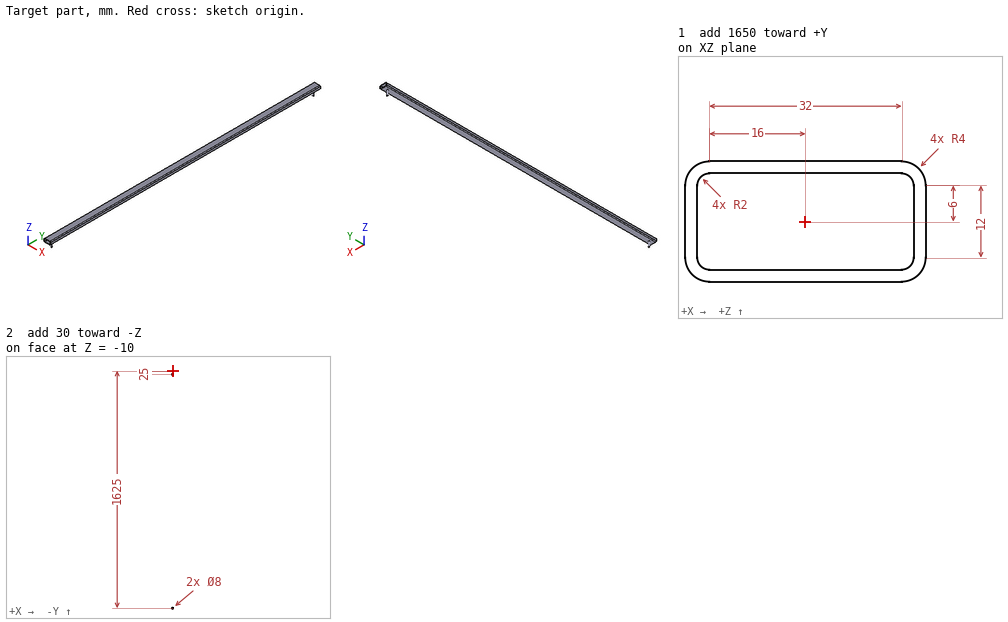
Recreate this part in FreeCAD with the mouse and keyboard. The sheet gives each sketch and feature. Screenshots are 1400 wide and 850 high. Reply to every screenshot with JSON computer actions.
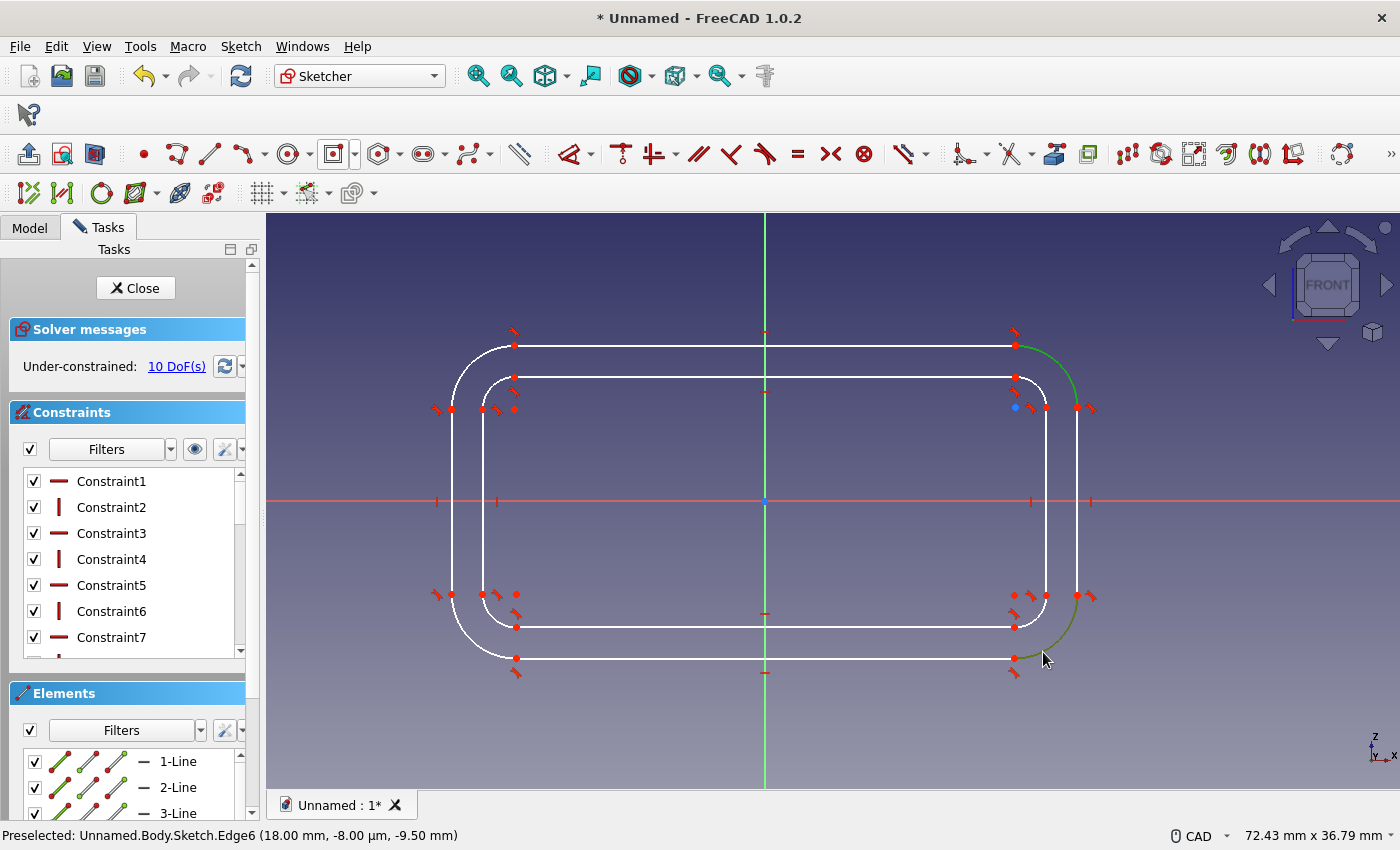
{"action": "left_click", "coordinate": [459, 623]}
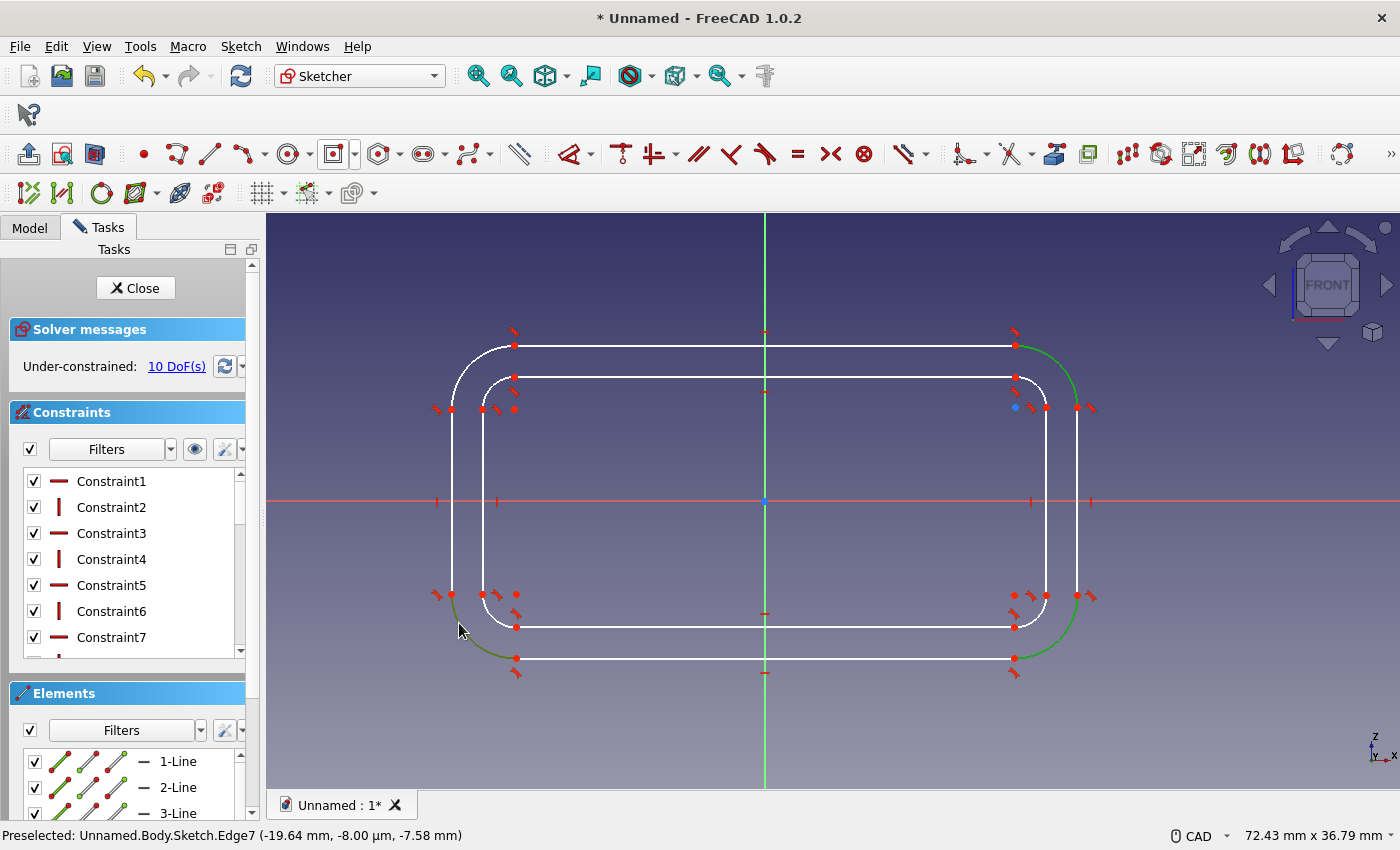
{"action": "left_click", "coordinate": [486, 353]}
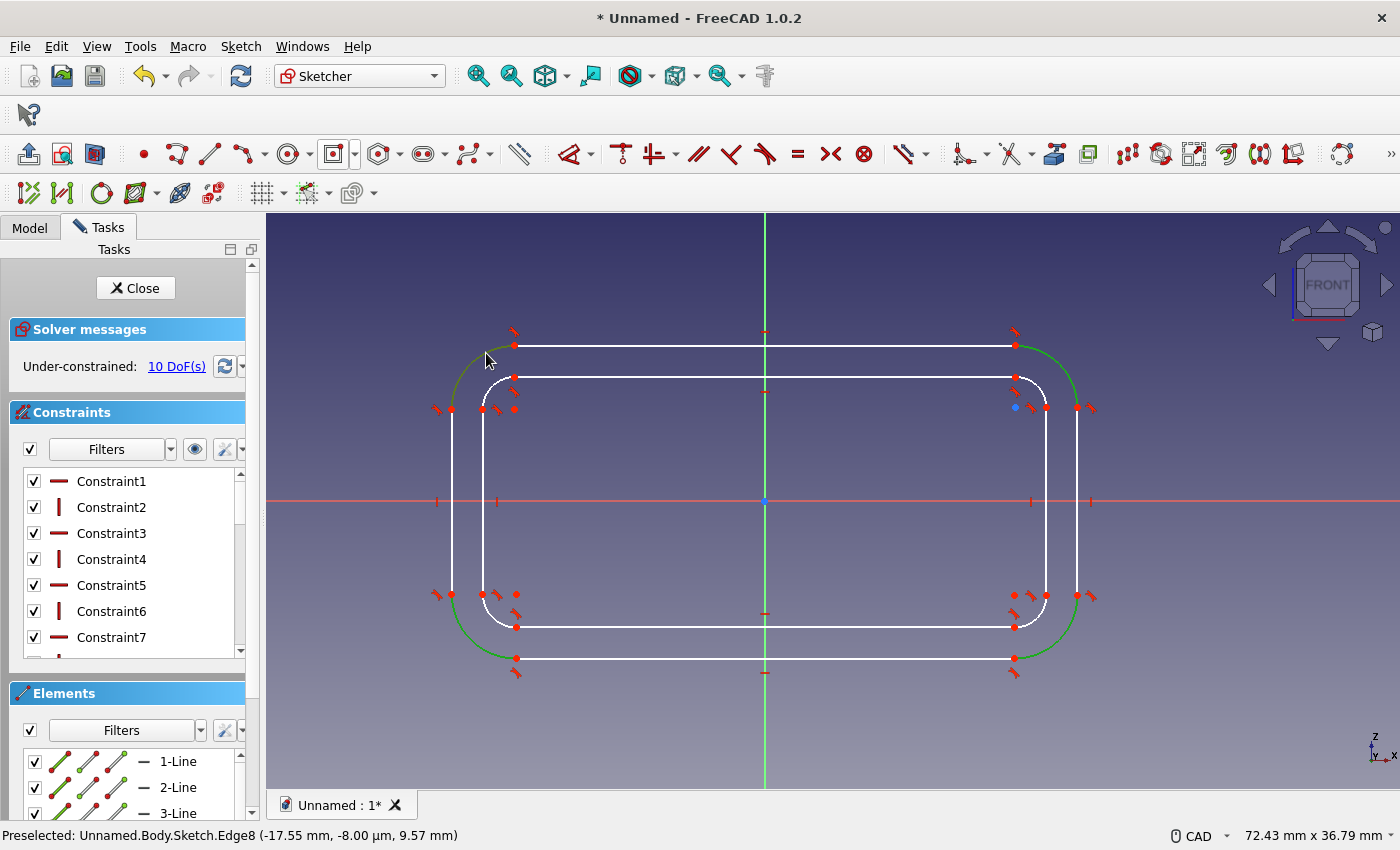
{"action": "key", "text": "e"}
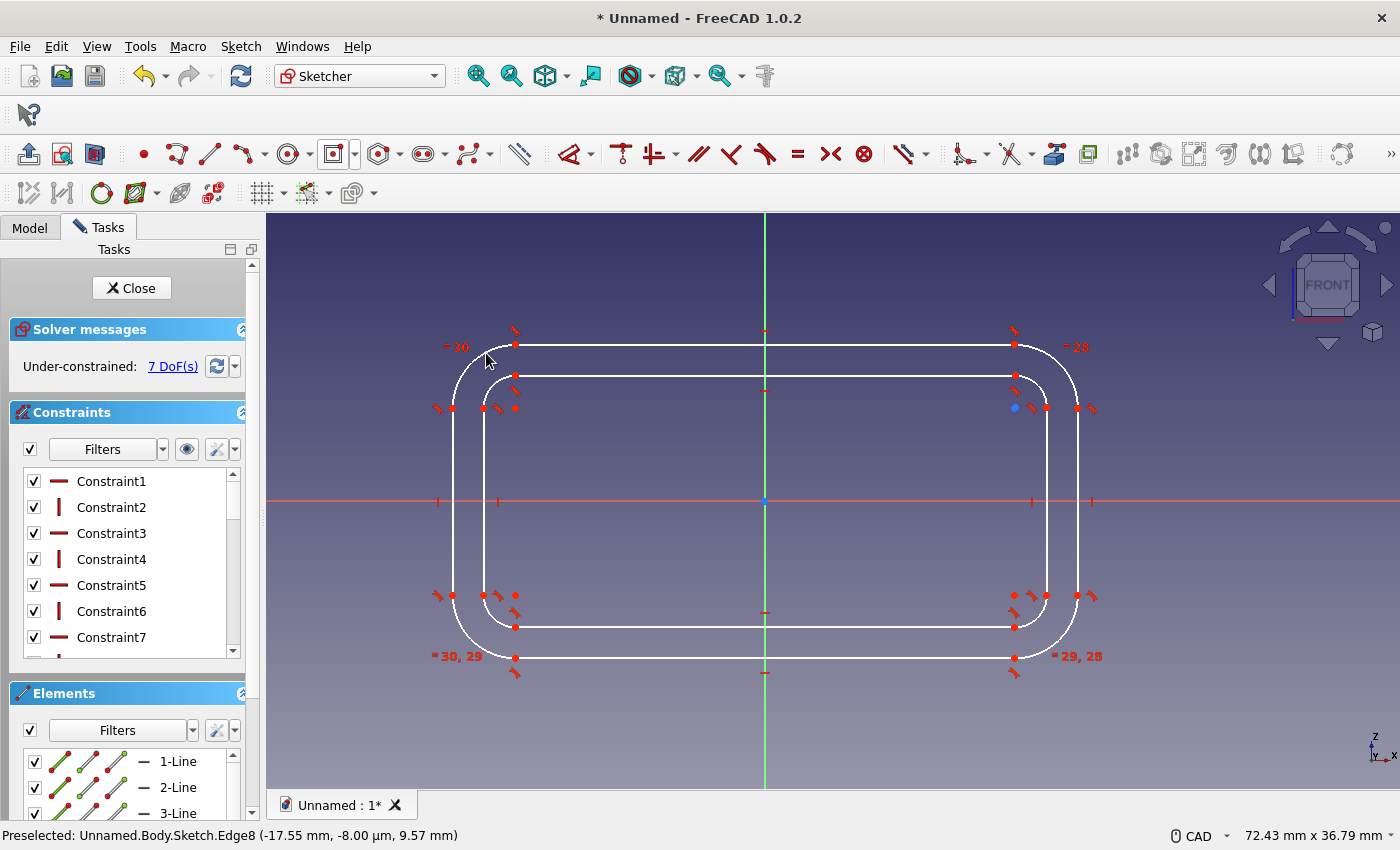
{"action": "left_click", "coordinate": [501, 379]}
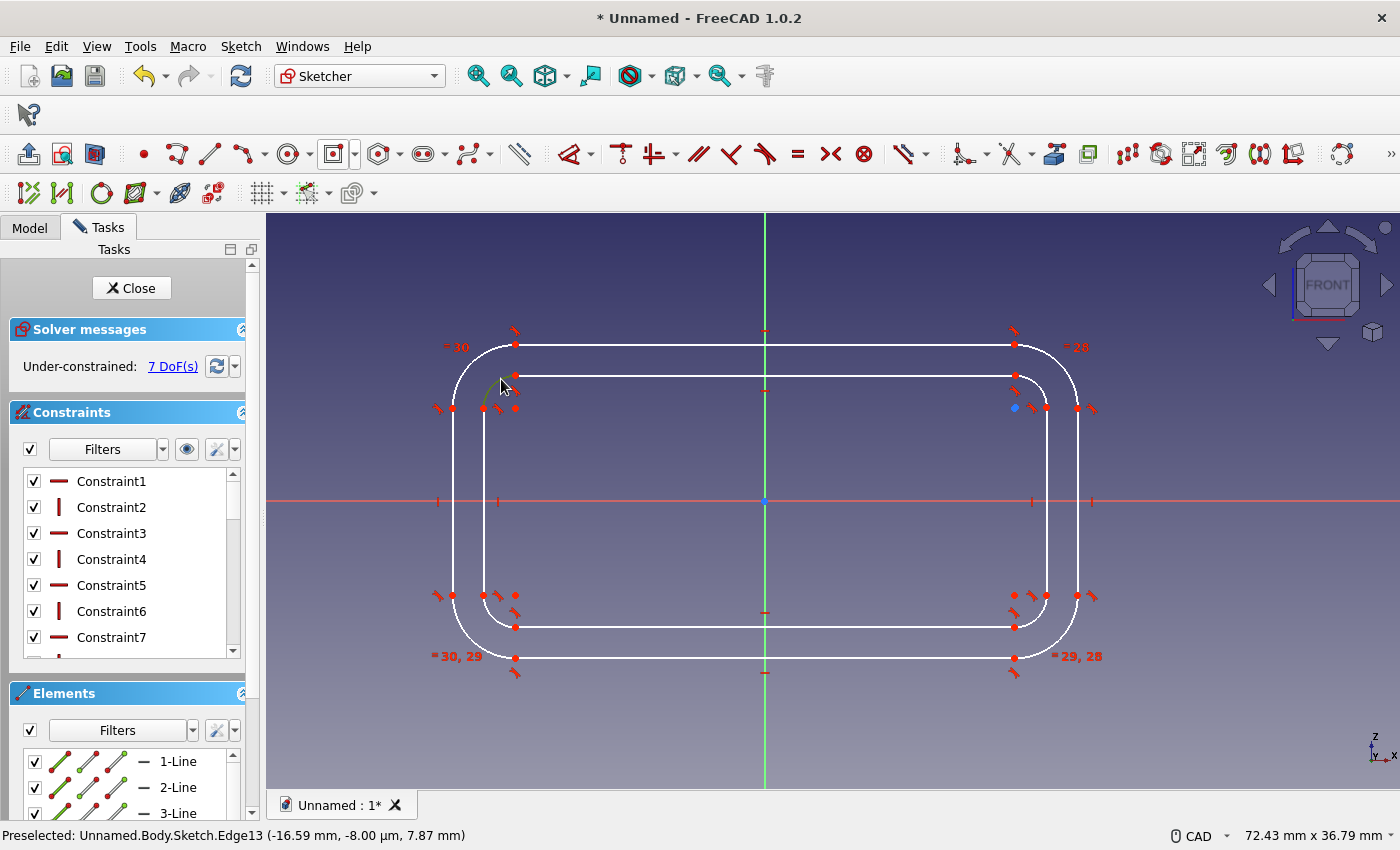
{"action": "left_click", "coordinate": [1043, 393]}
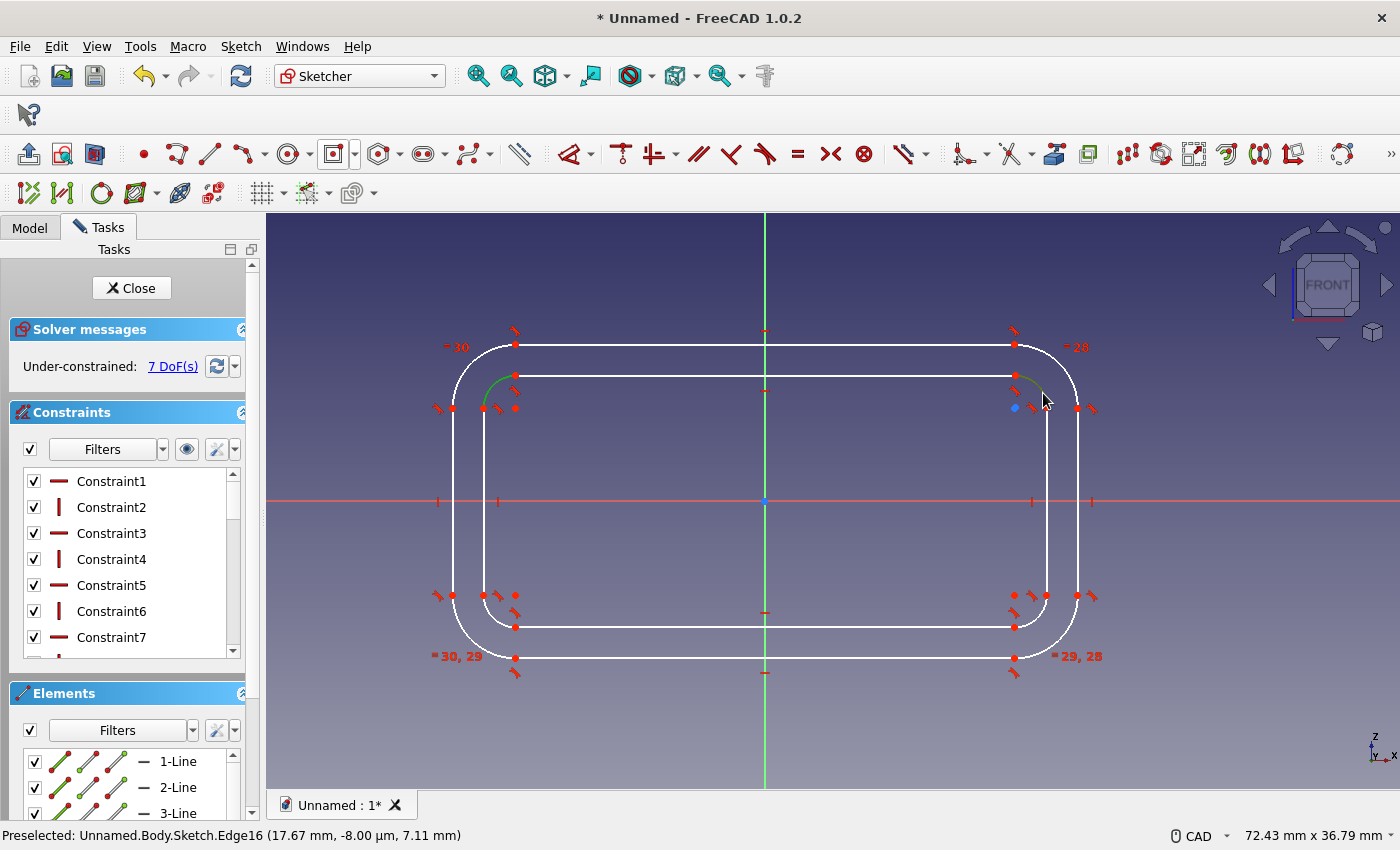
{"action": "left_click", "coordinate": [798, 154]}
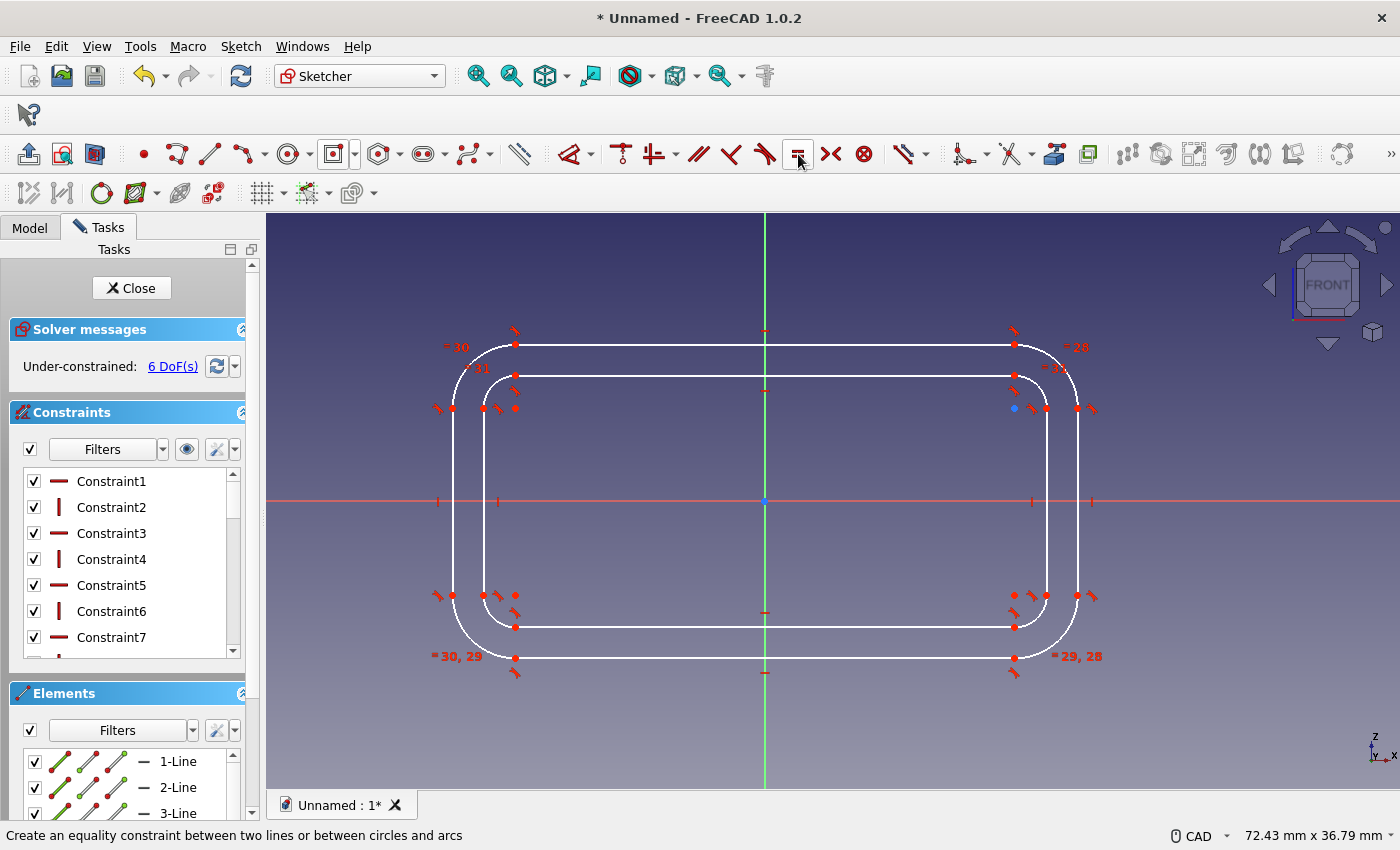
{"action": "left_click", "coordinate": [568, 154]}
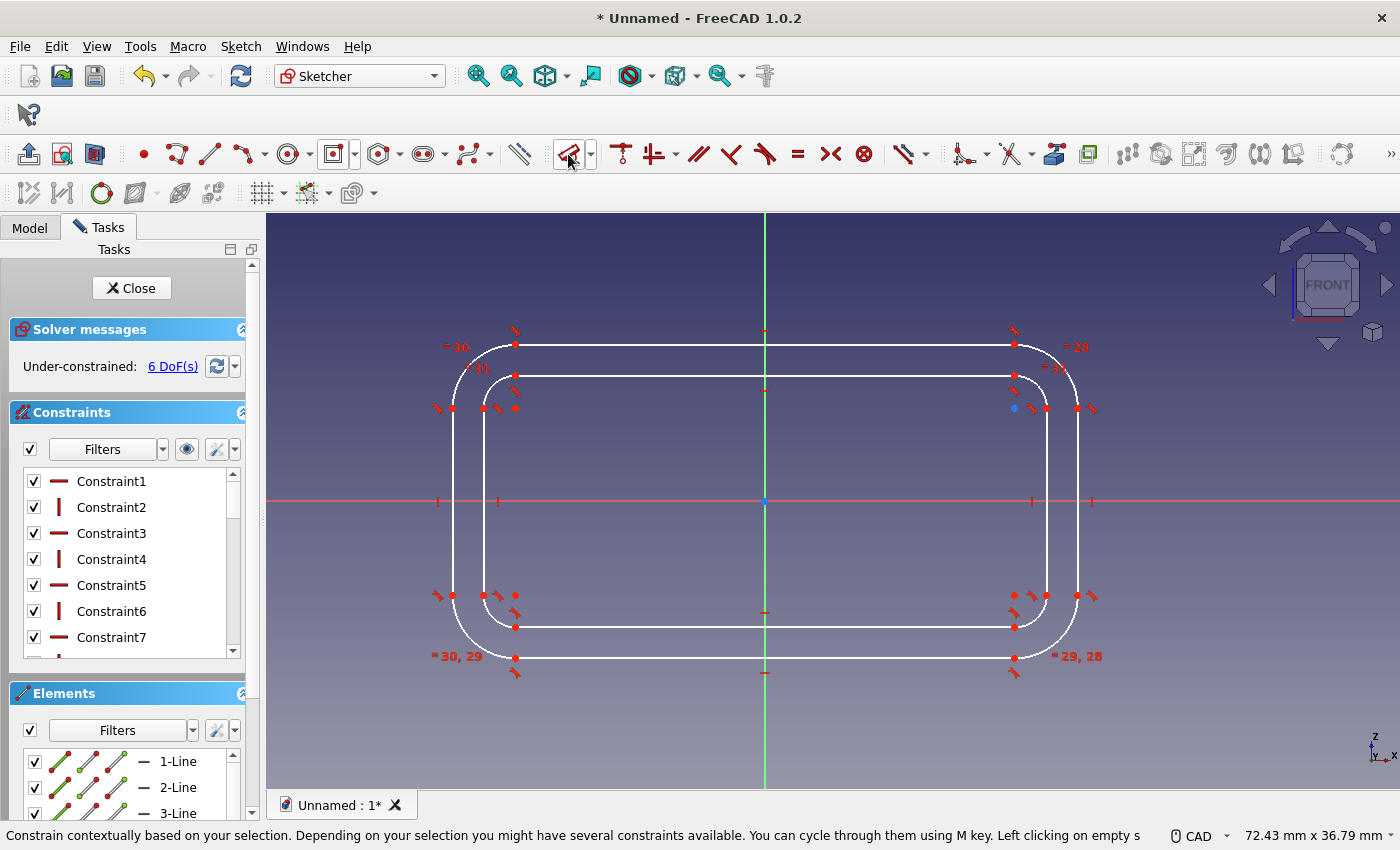
{"action": "left_click", "coordinate": [1071, 379]}
{"action": "left_click", "coordinate": [1099, 364]}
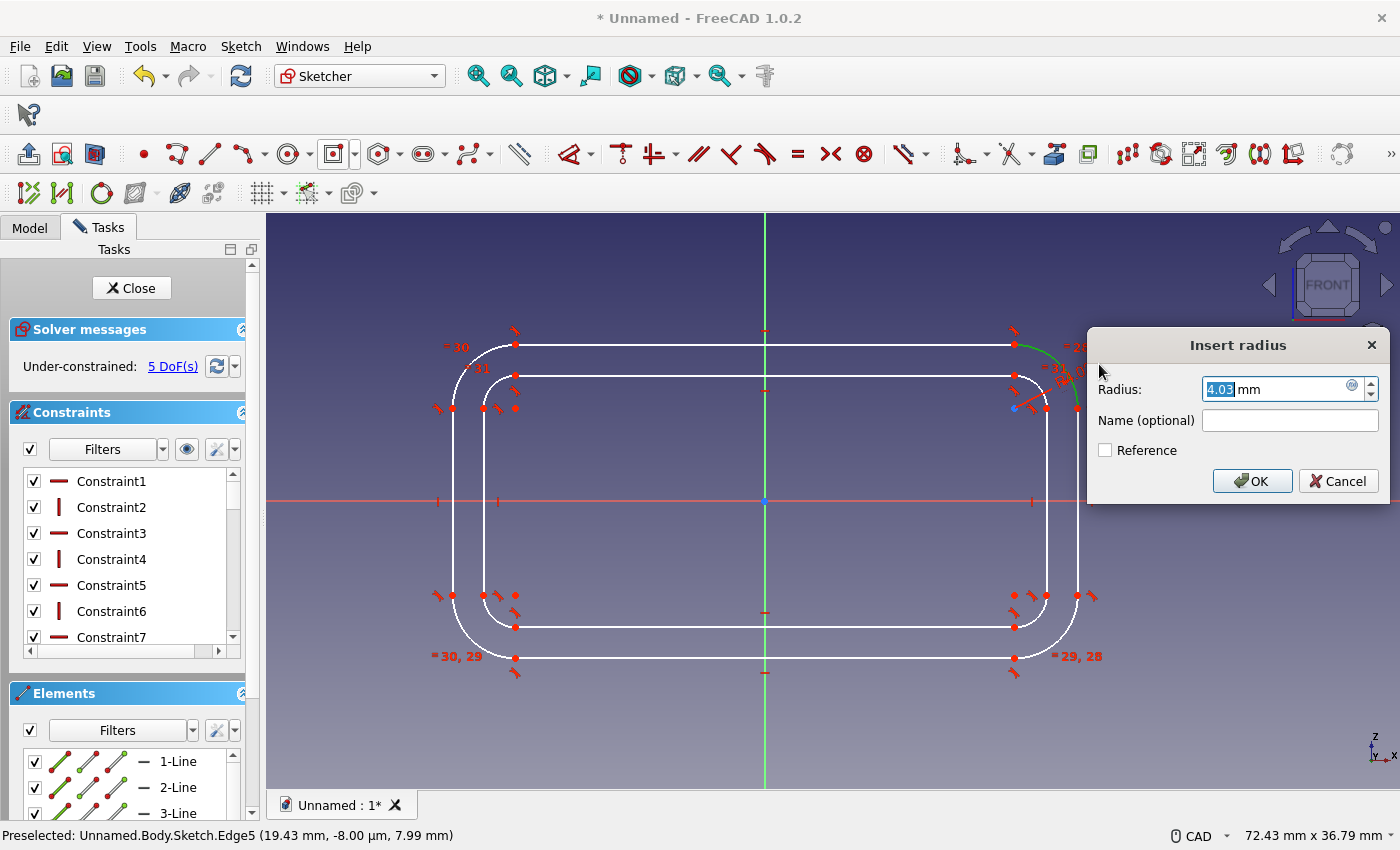
{"action": "type", "text": "4"}
{"action": "key", "text": "Return"}